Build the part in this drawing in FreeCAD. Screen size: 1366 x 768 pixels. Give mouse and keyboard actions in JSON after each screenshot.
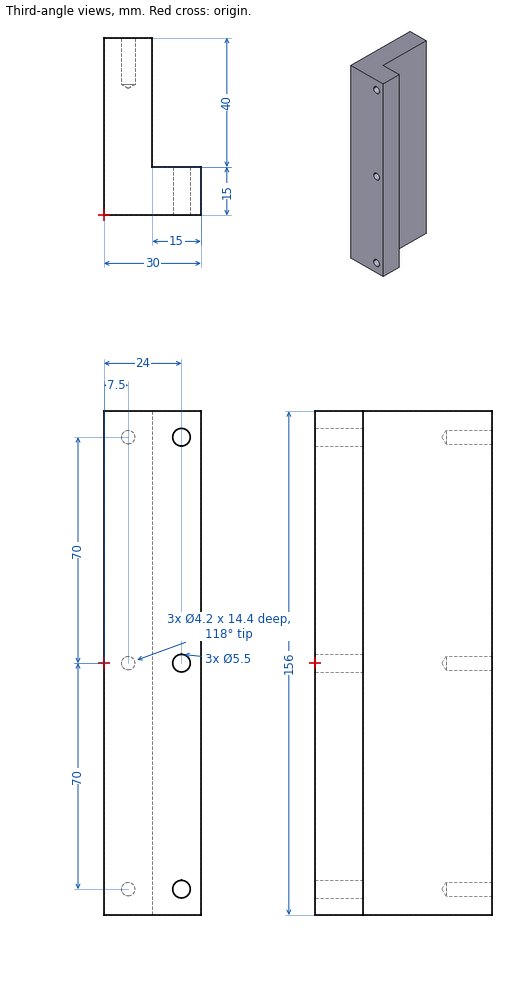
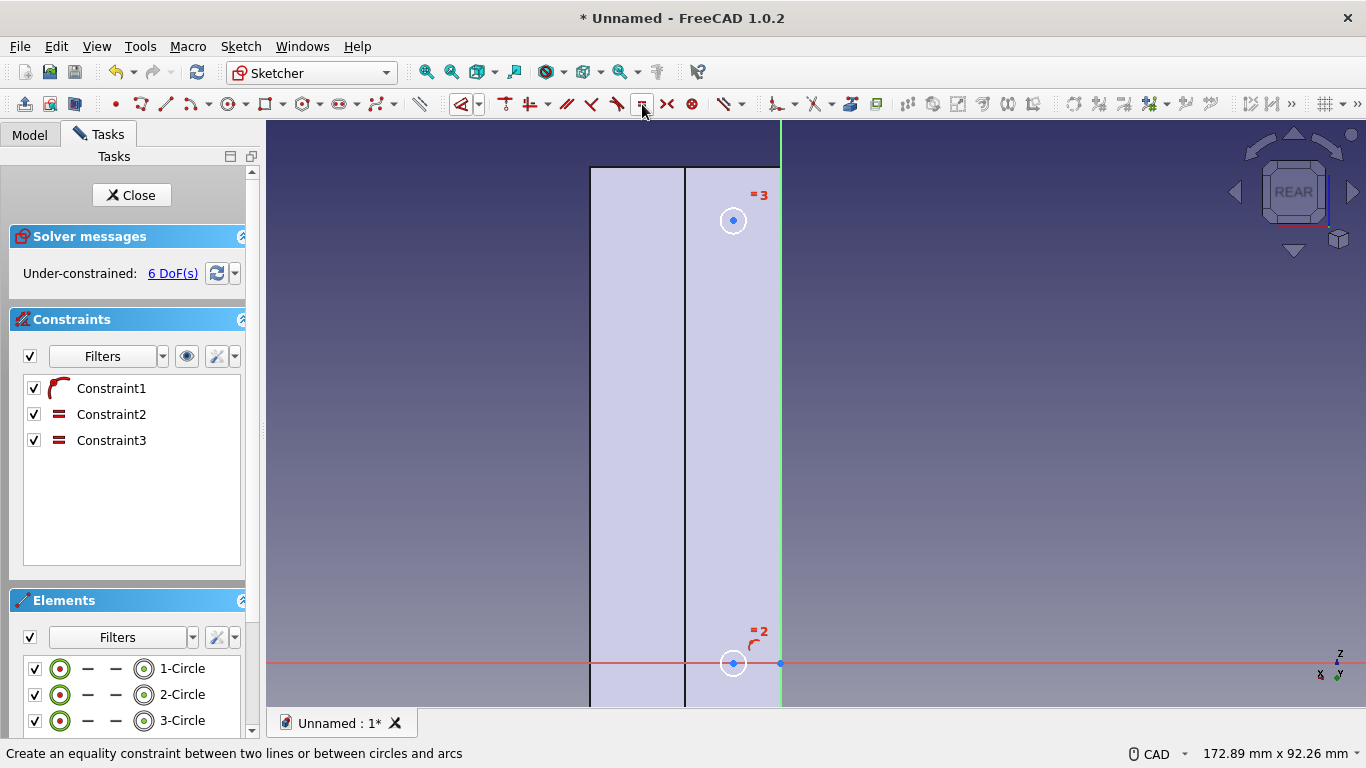
{"action": "left_click", "coordinate": [733, 663]}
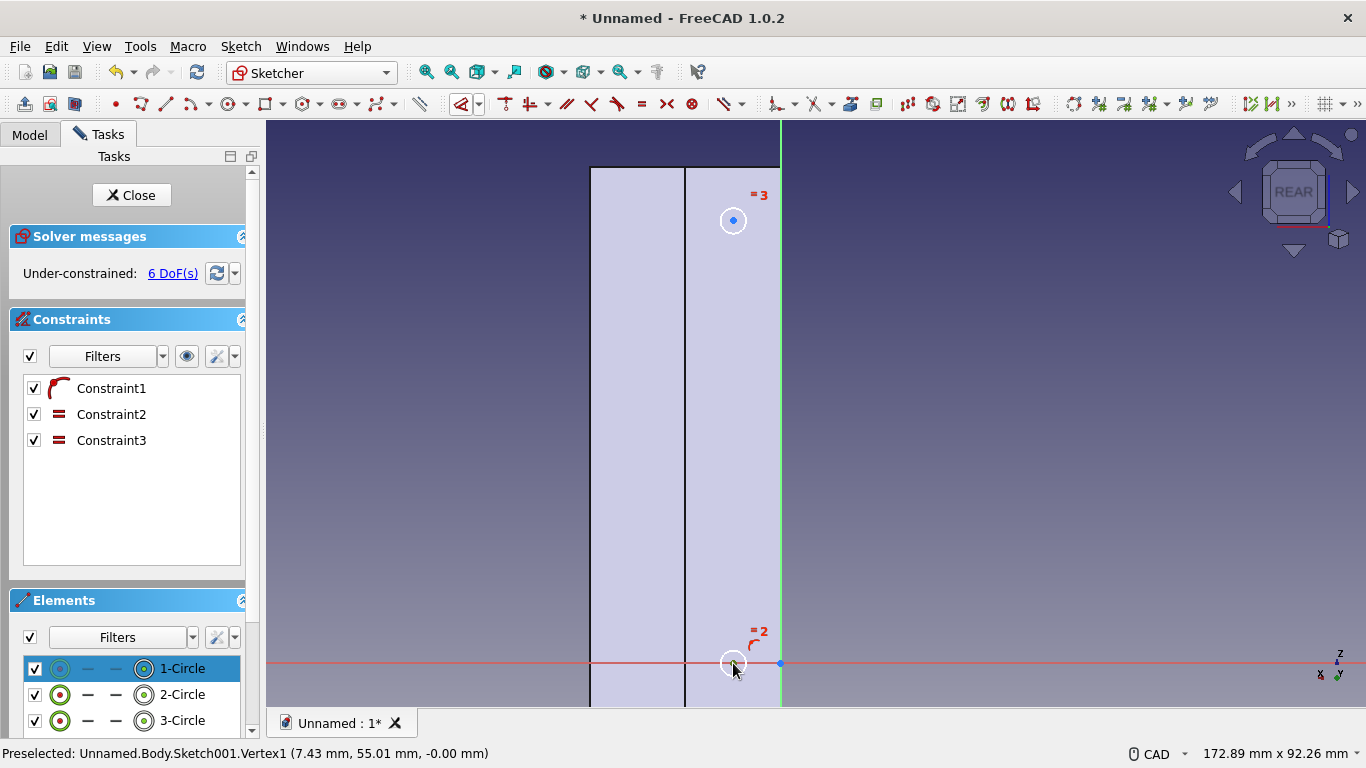
{"action": "scroll", "coordinate": [745, 210], "scroll_direction": "down", "scroll_amount": 4}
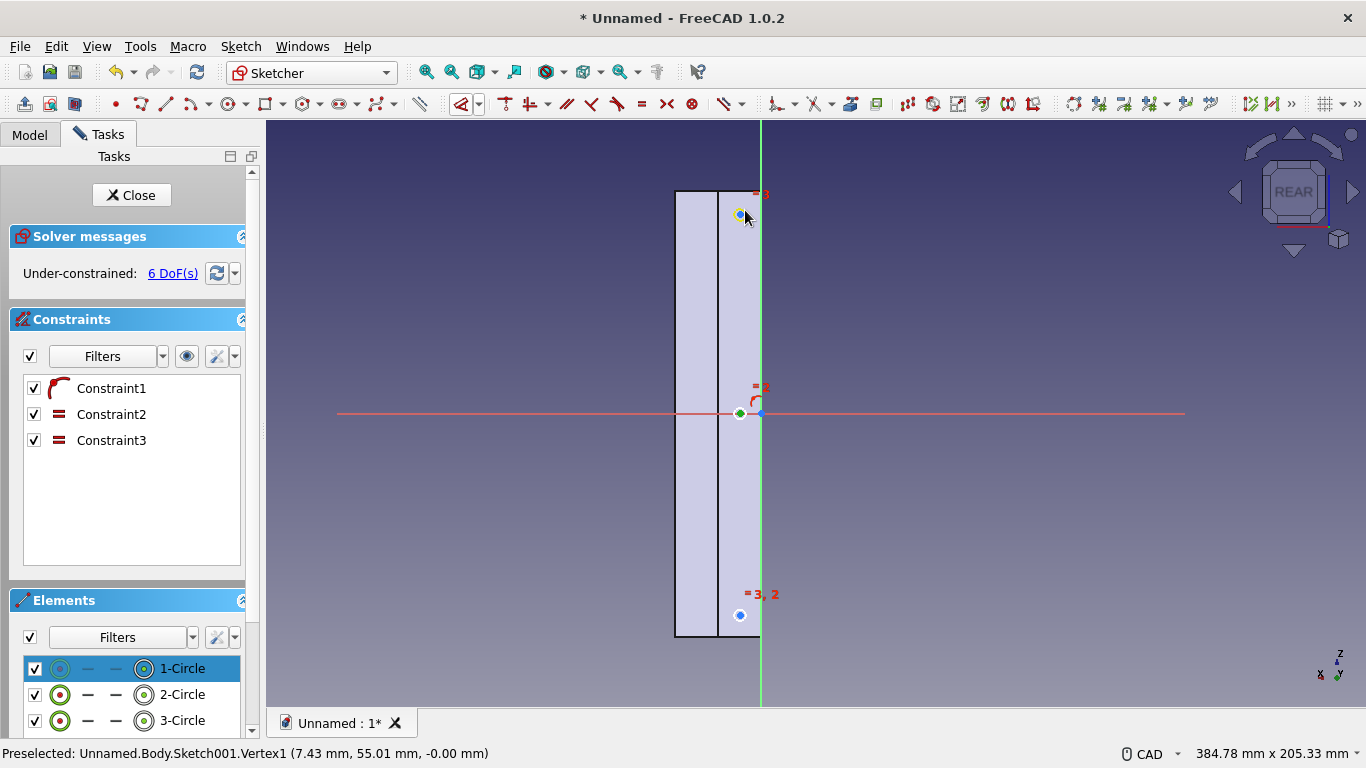
{"action": "left_click", "coordinate": [740, 615]}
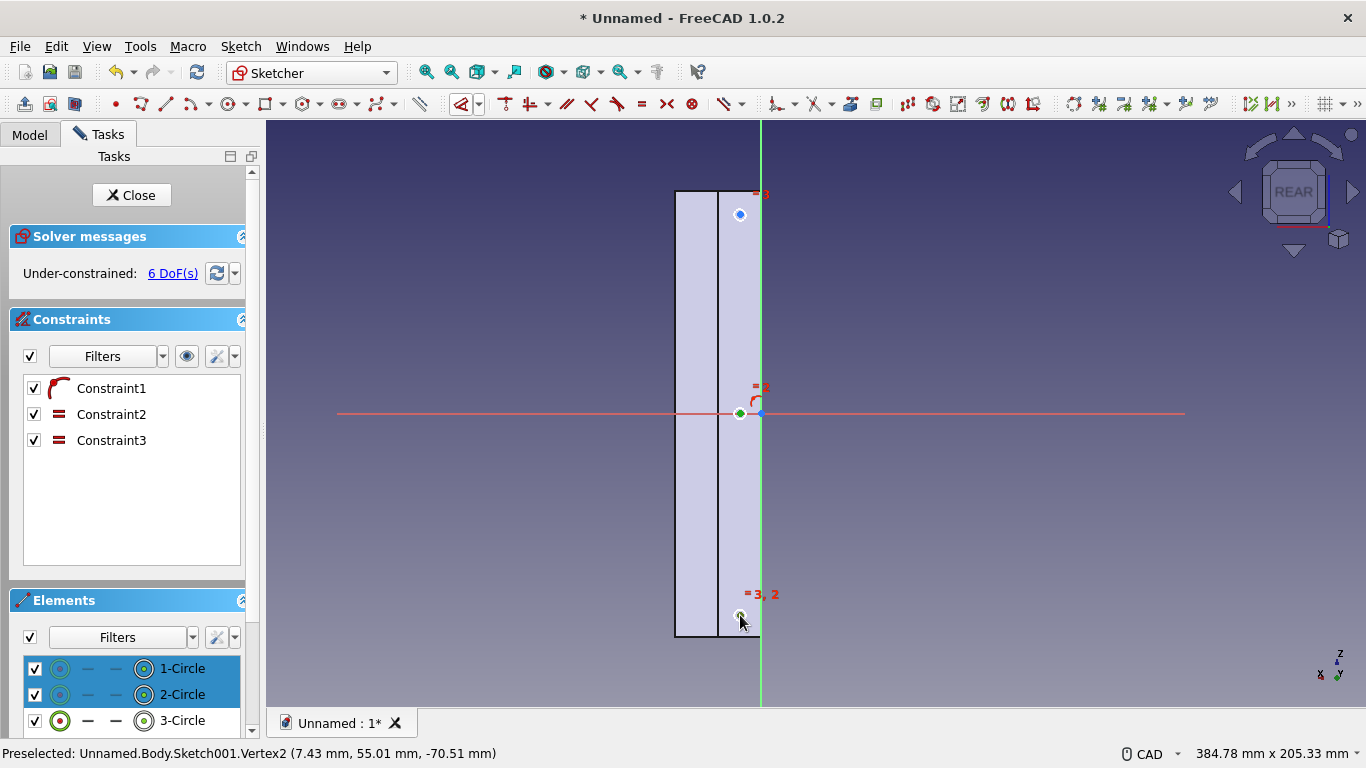
{"action": "key", "text": "v"}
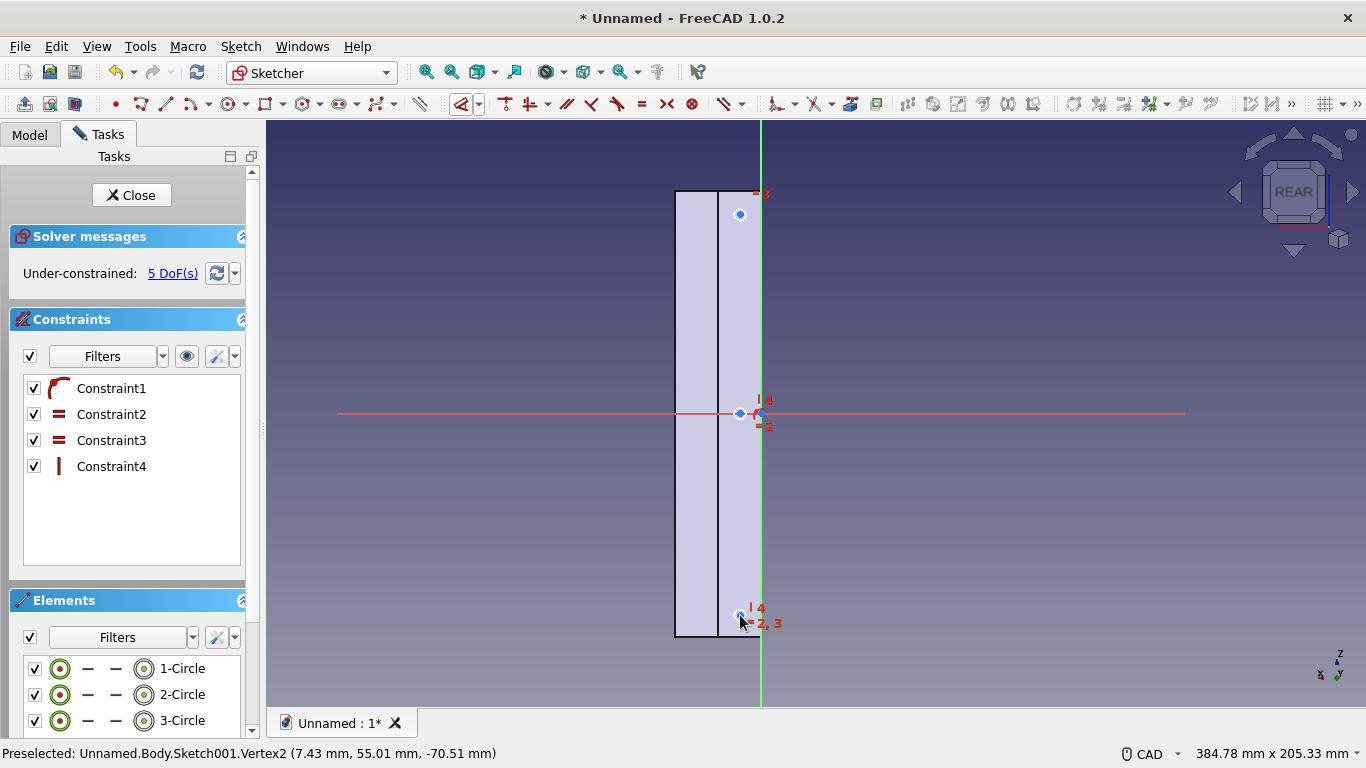
{"action": "left_click", "coordinate": [740, 414]}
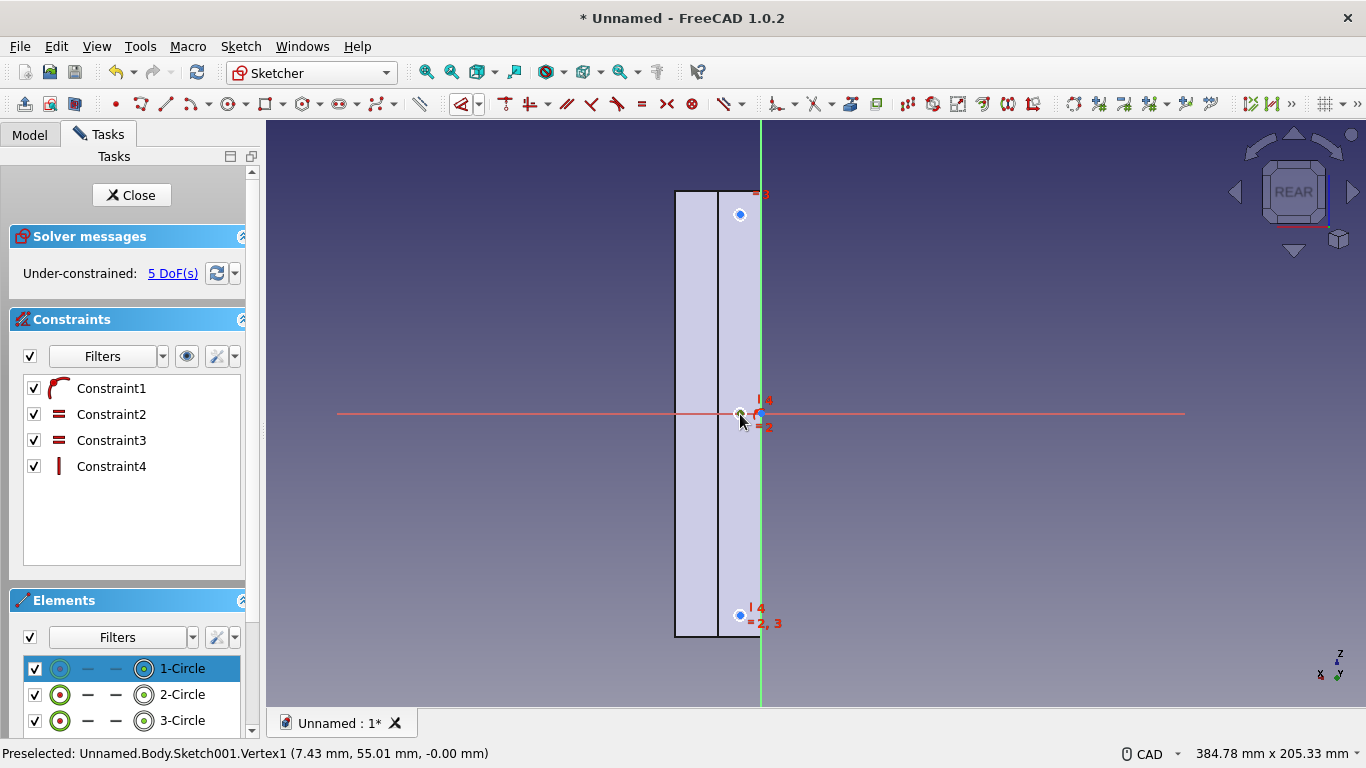
{"action": "left_click", "coordinate": [740, 215]}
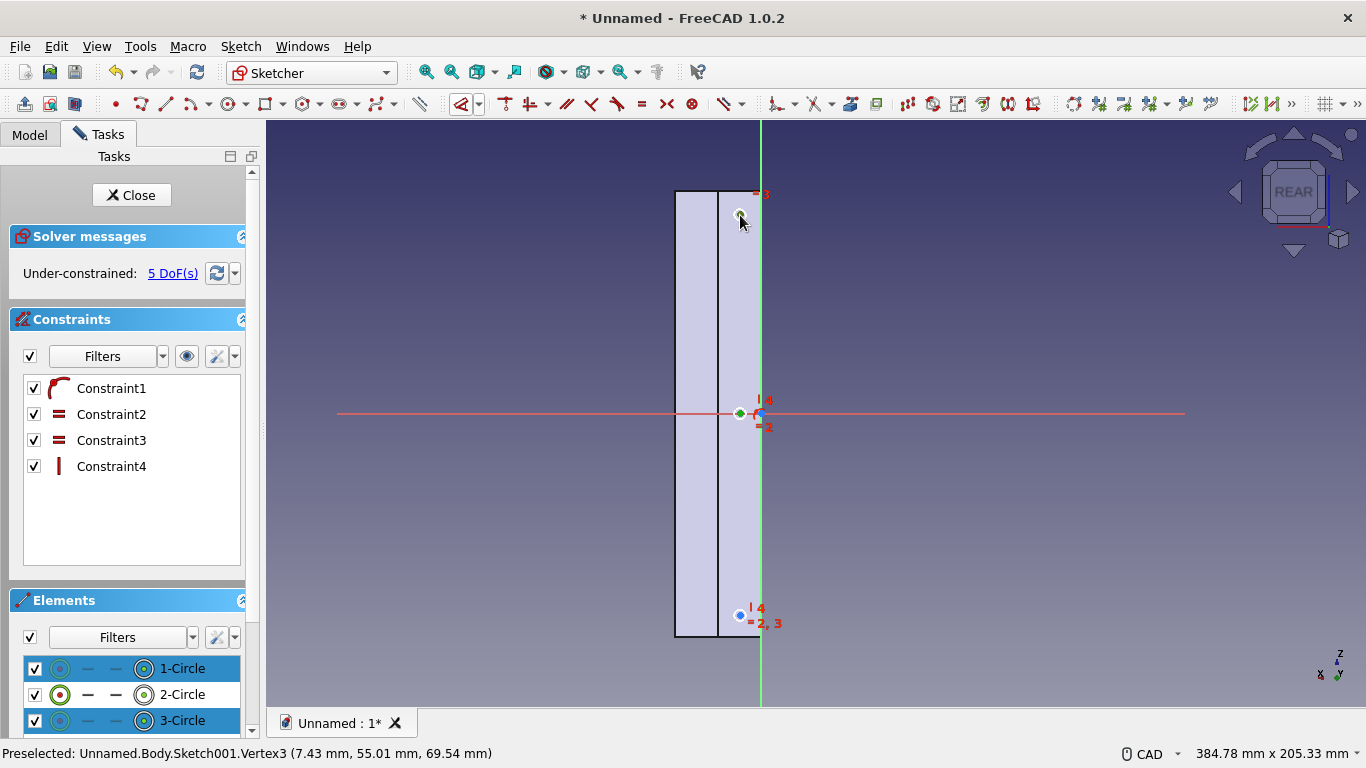
{"action": "key", "text": "v"}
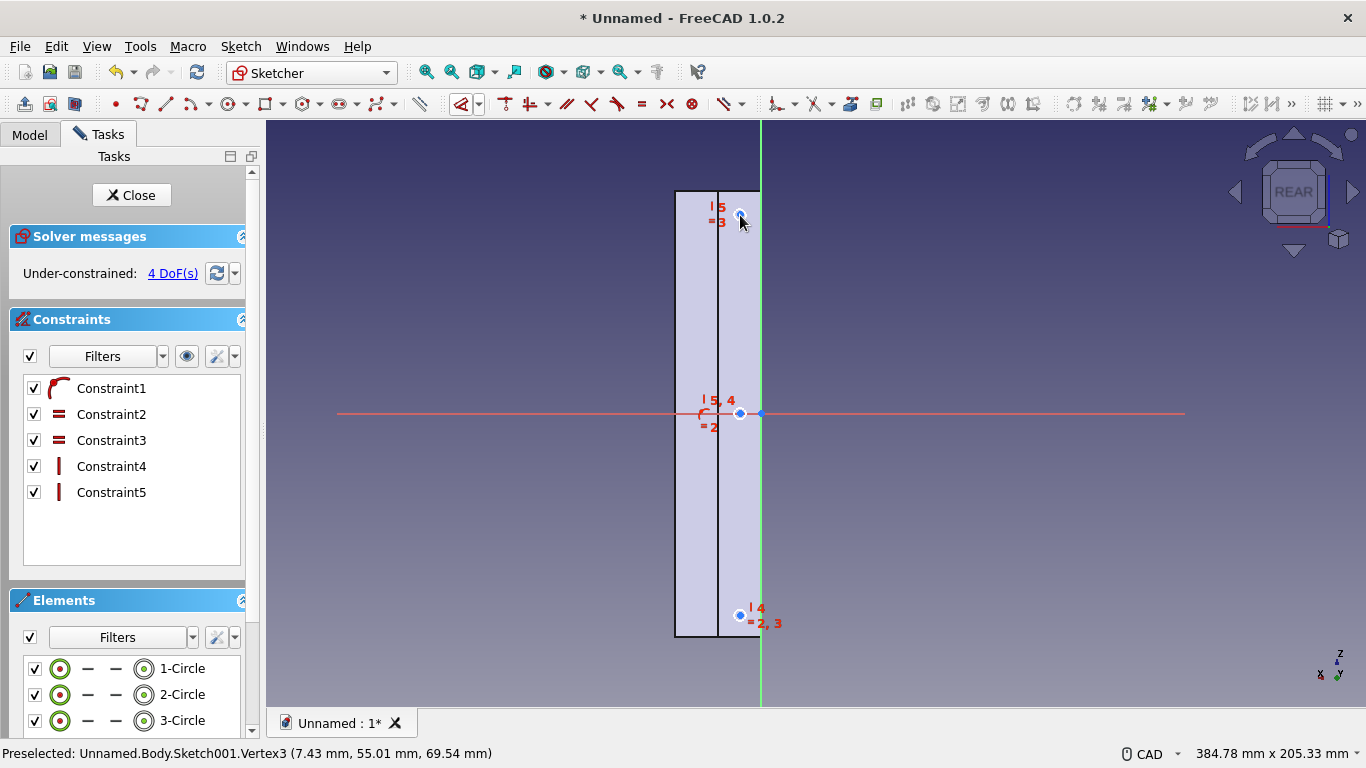
{"action": "scroll", "coordinate": [734, 414], "scroll_direction": "up", "scroll_amount": 6}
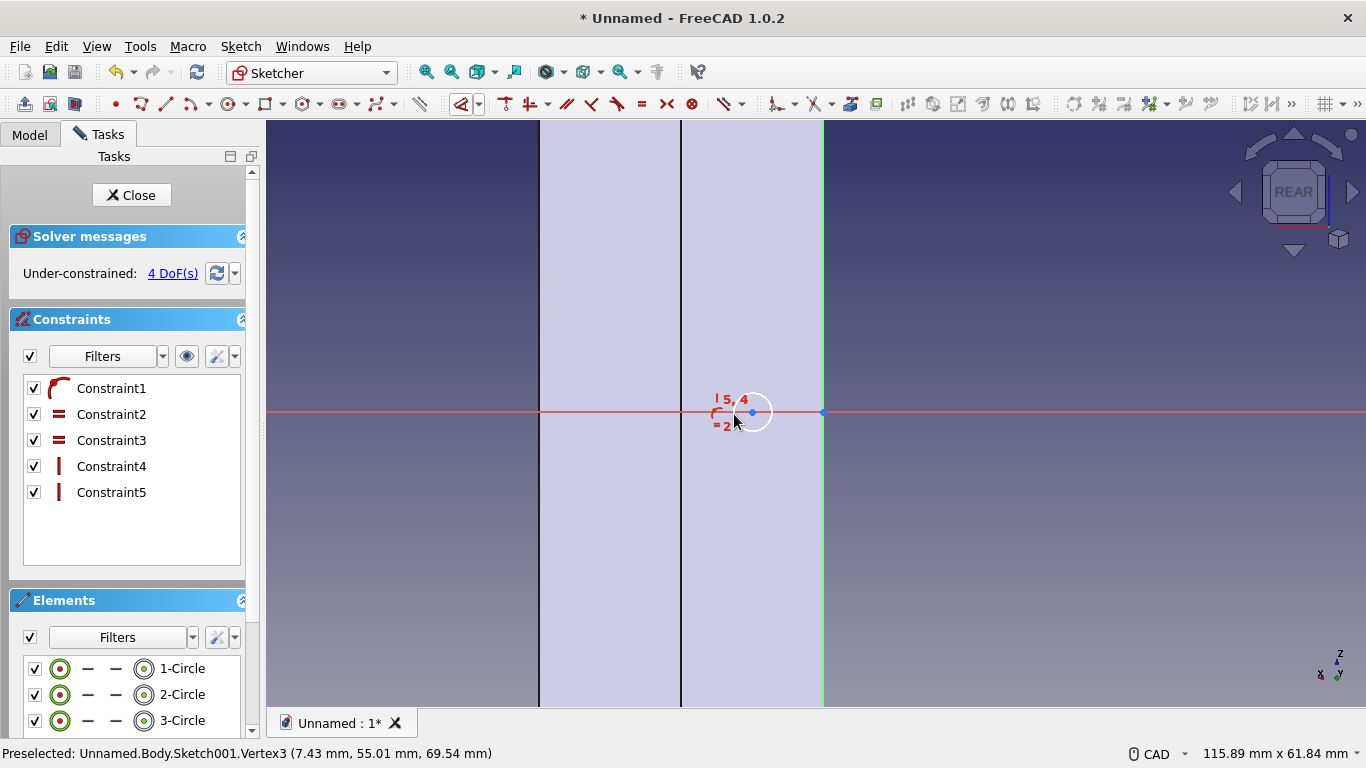
{"action": "left_click", "coordinate": [772, 413]}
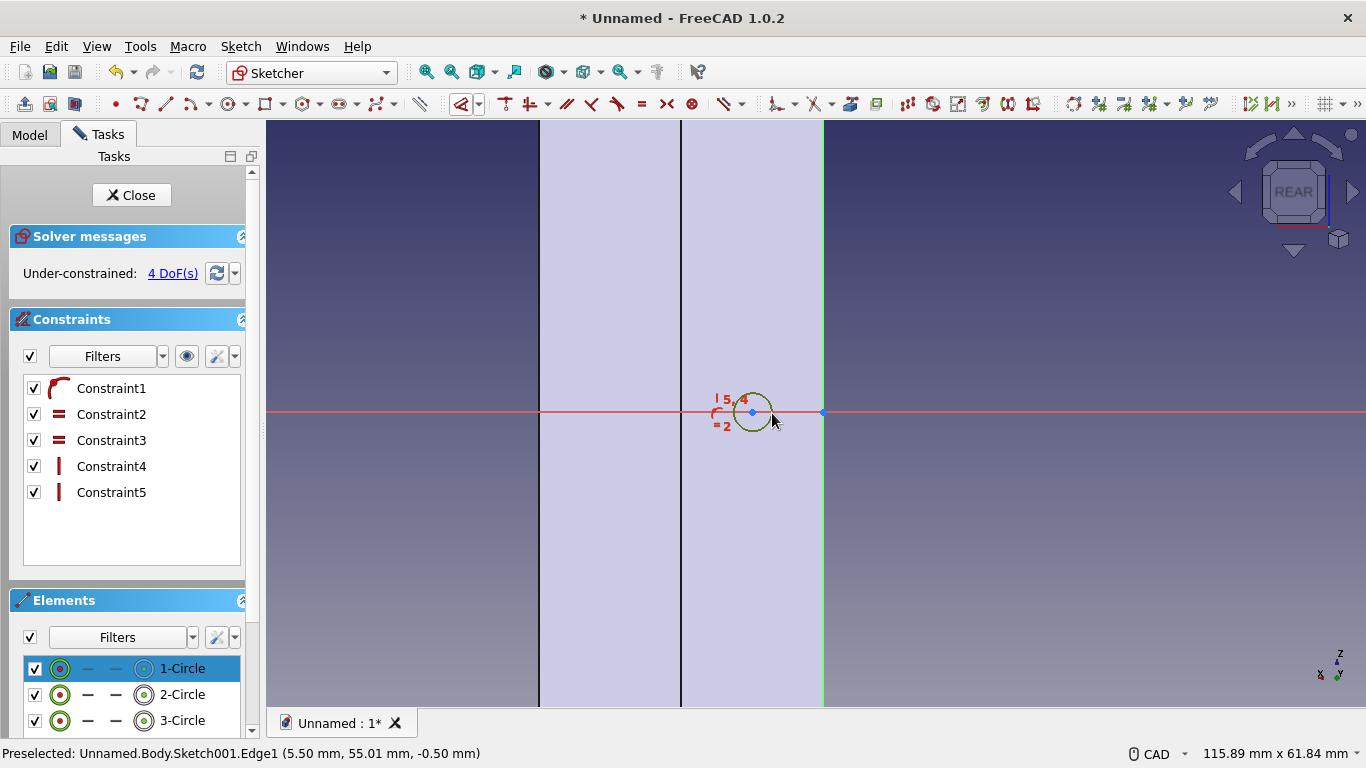
{"action": "key", "text": "k o"}